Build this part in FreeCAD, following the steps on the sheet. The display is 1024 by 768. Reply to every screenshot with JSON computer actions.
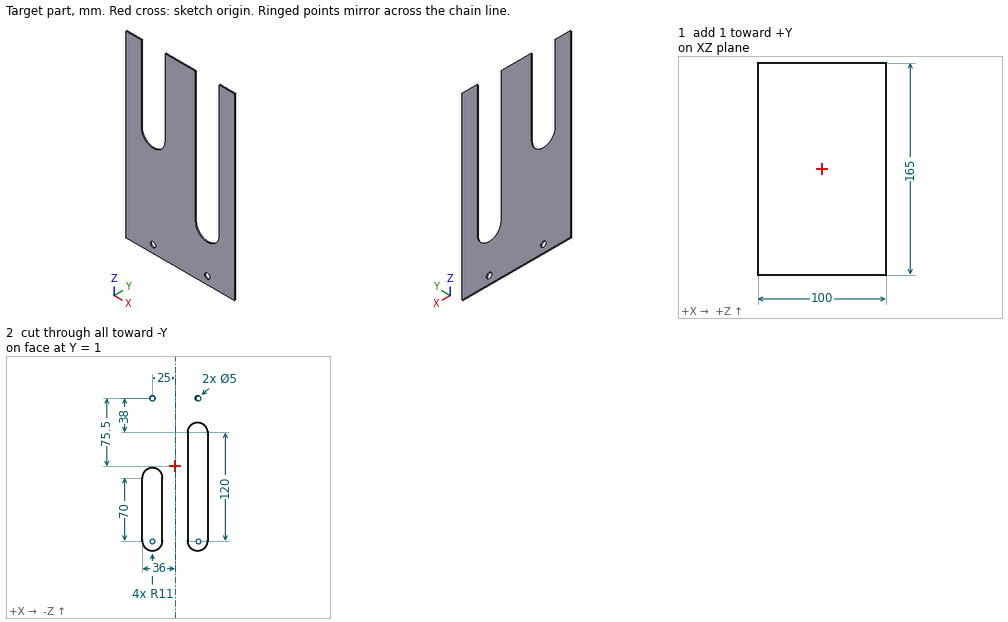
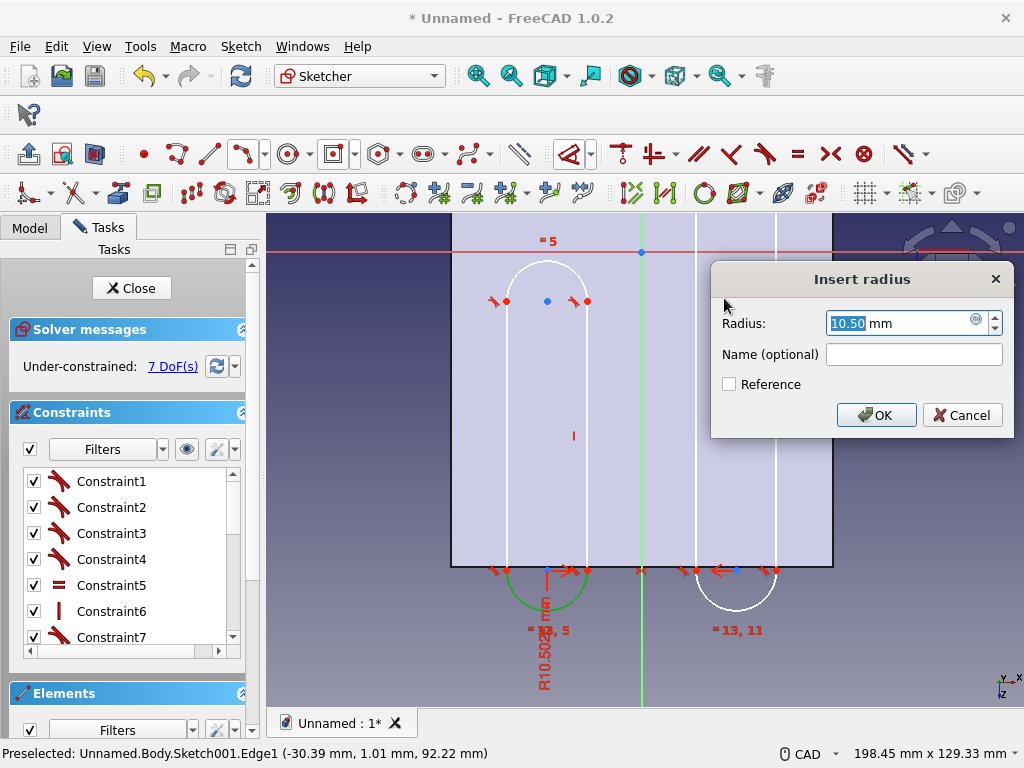
{"action": "type", "text": "11"}
{"action": "key", "text": "Return"}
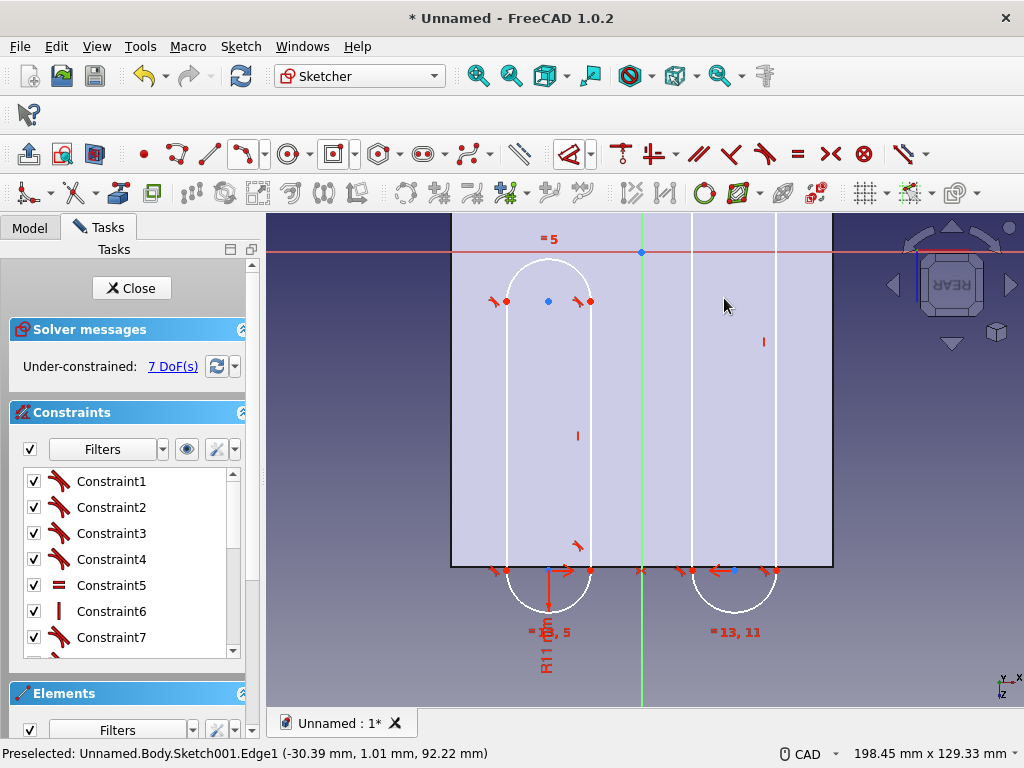
{"action": "scroll", "coordinate": [523, 605], "scroll_direction": "down", "scroll_amount": 4}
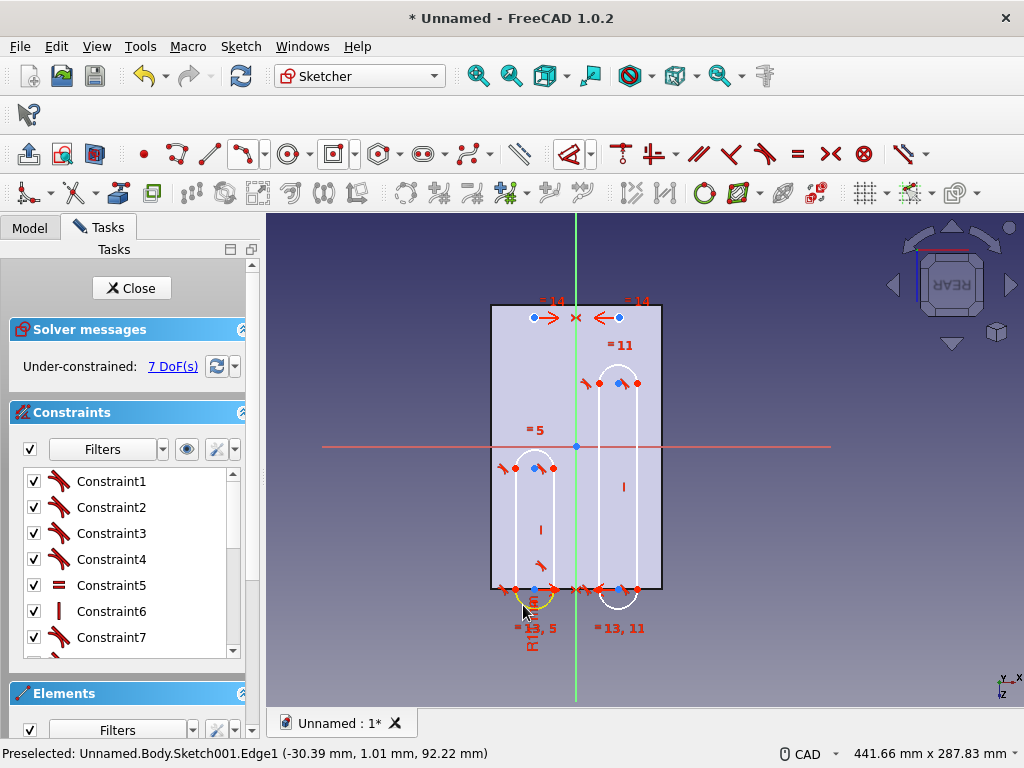
{"action": "scroll", "coordinate": [537, 315], "scroll_direction": "up", "scroll_amount": 8}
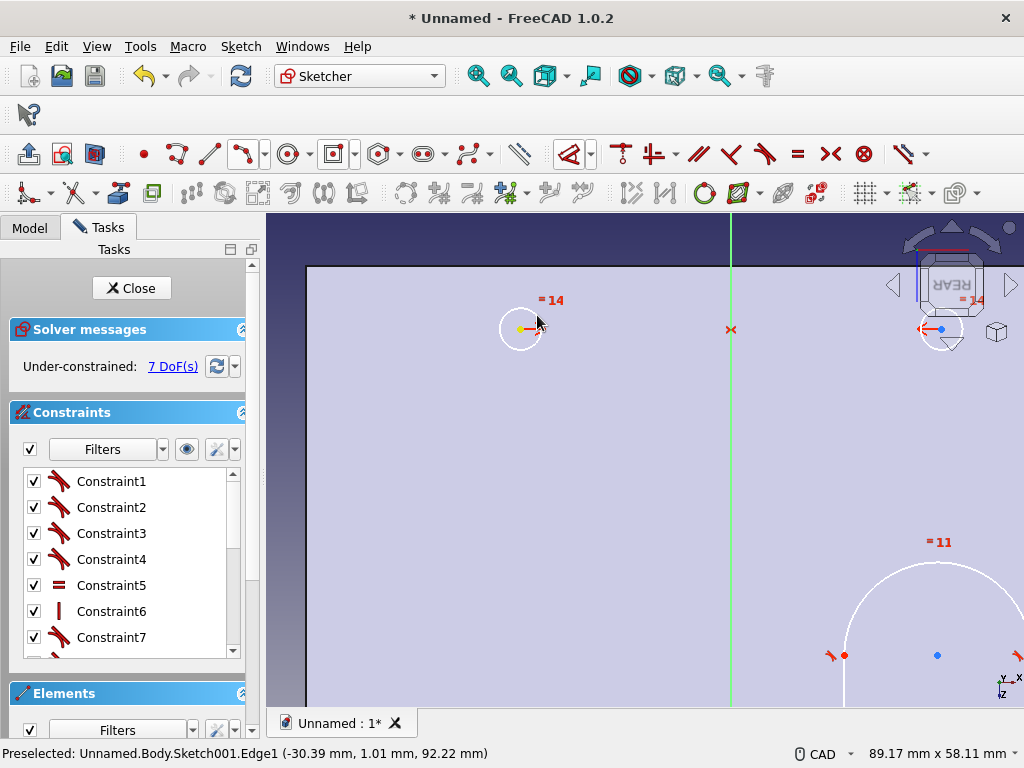
{"action": "left_click", "coordinate": [535, 314]}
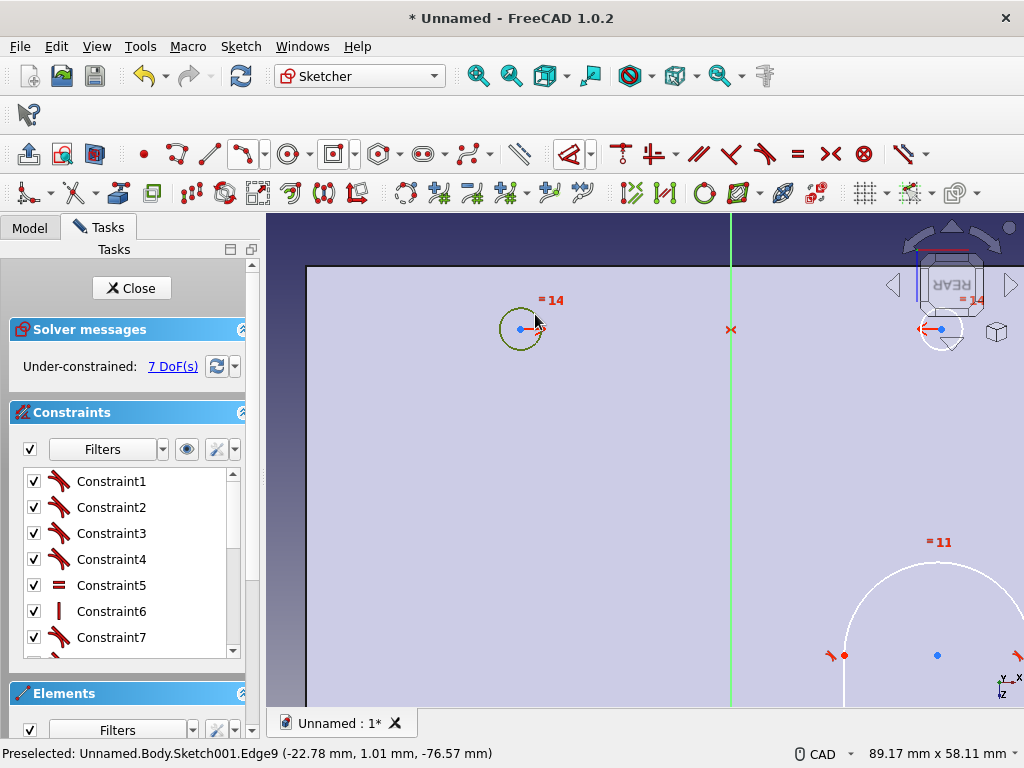
{"action": "key", "text": "k o"}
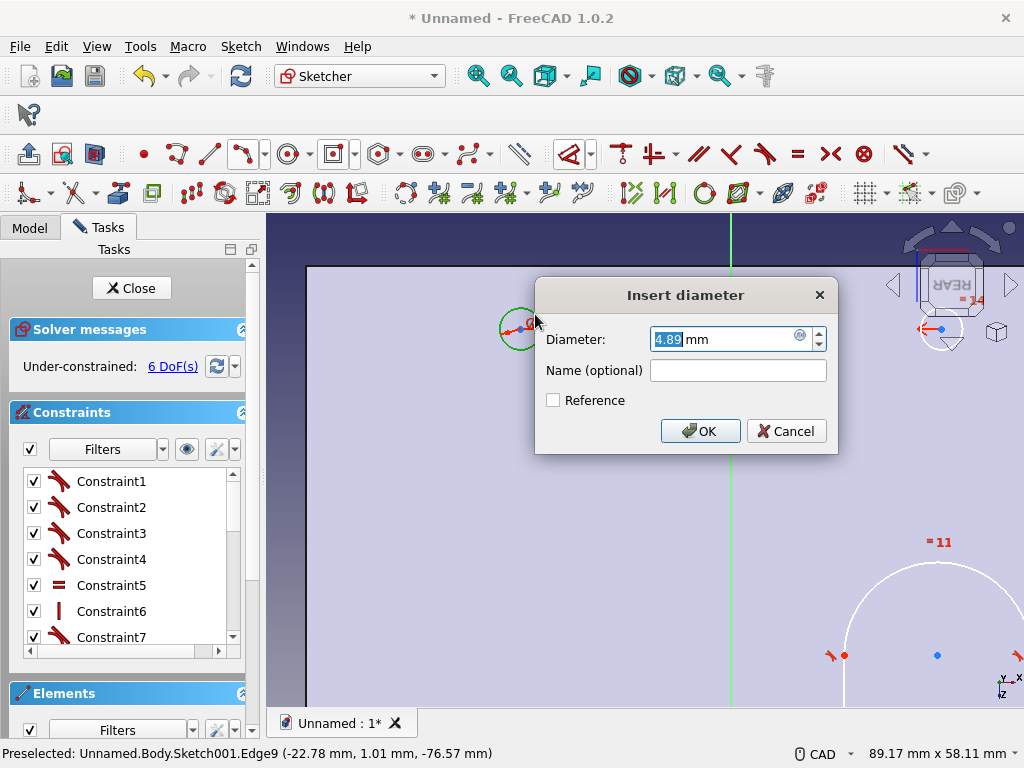
{"action": "type", "text": "5"}
{"action": "key", "text": "Return"}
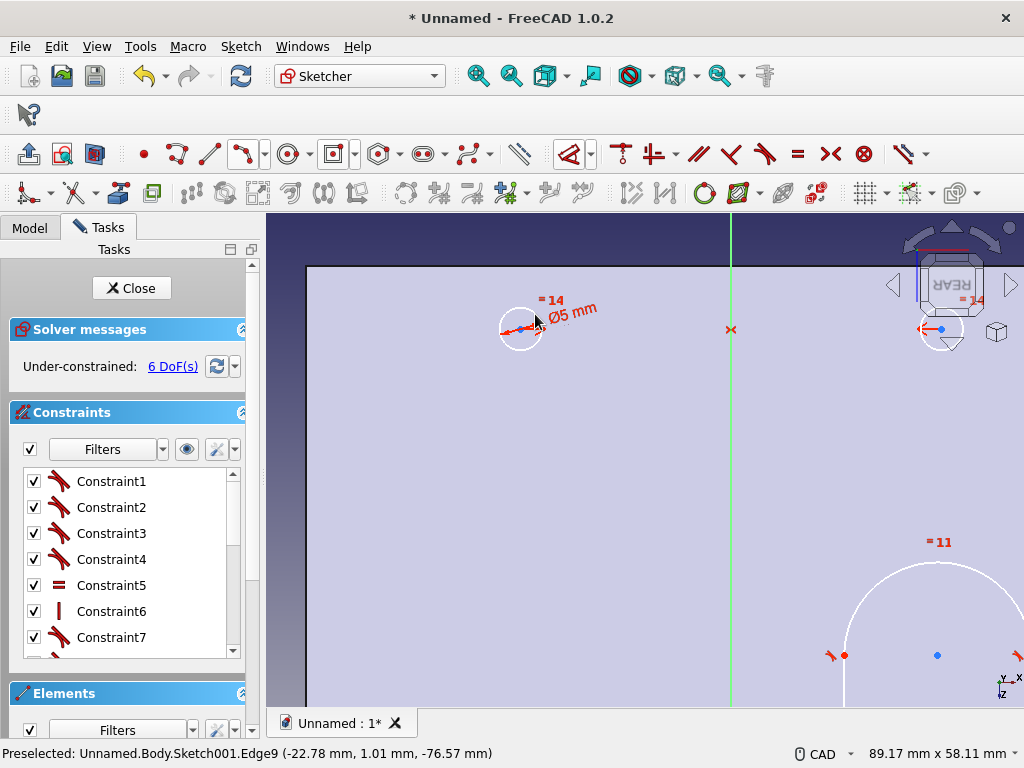
{"action": "scroll", "coordinate": [537, 315], "scroll_direction": "down", "scroll_amount": 8}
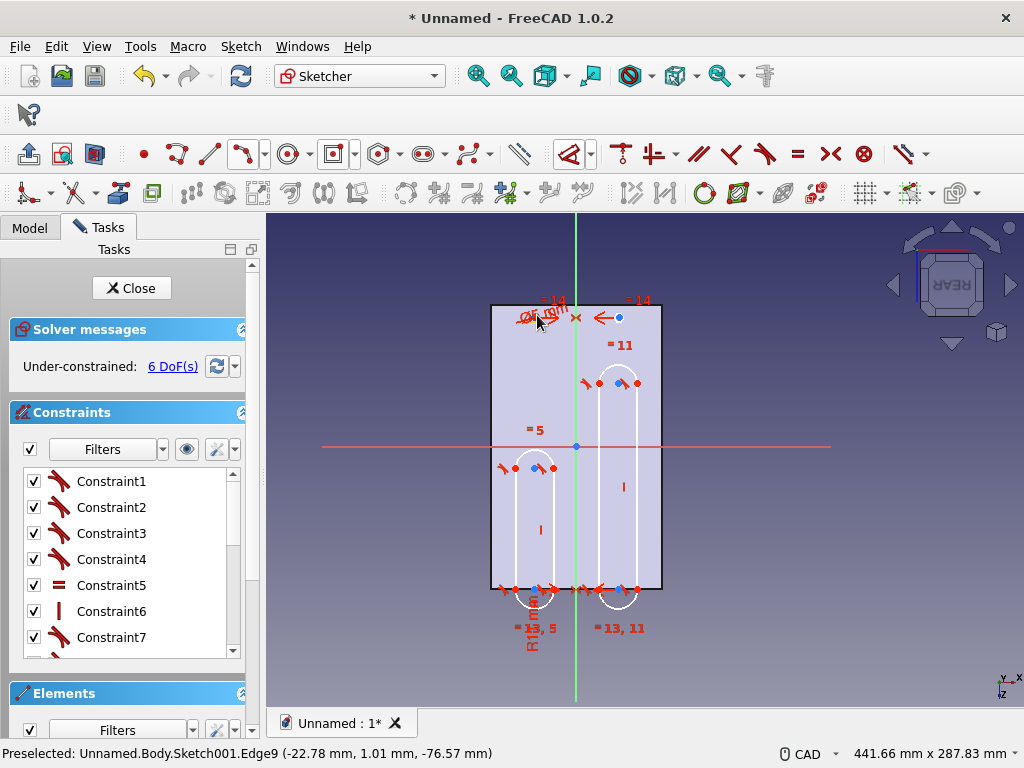
{"action": "left_click", "coordinate": [516, 554]}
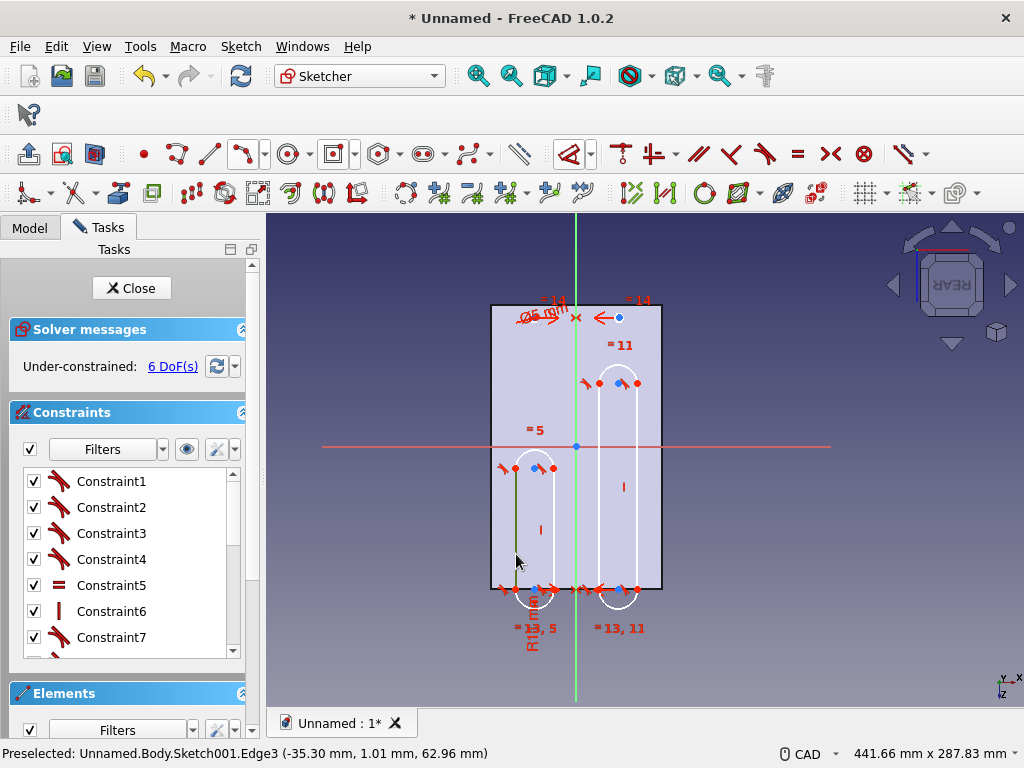
{"action": "key", "text": "i"}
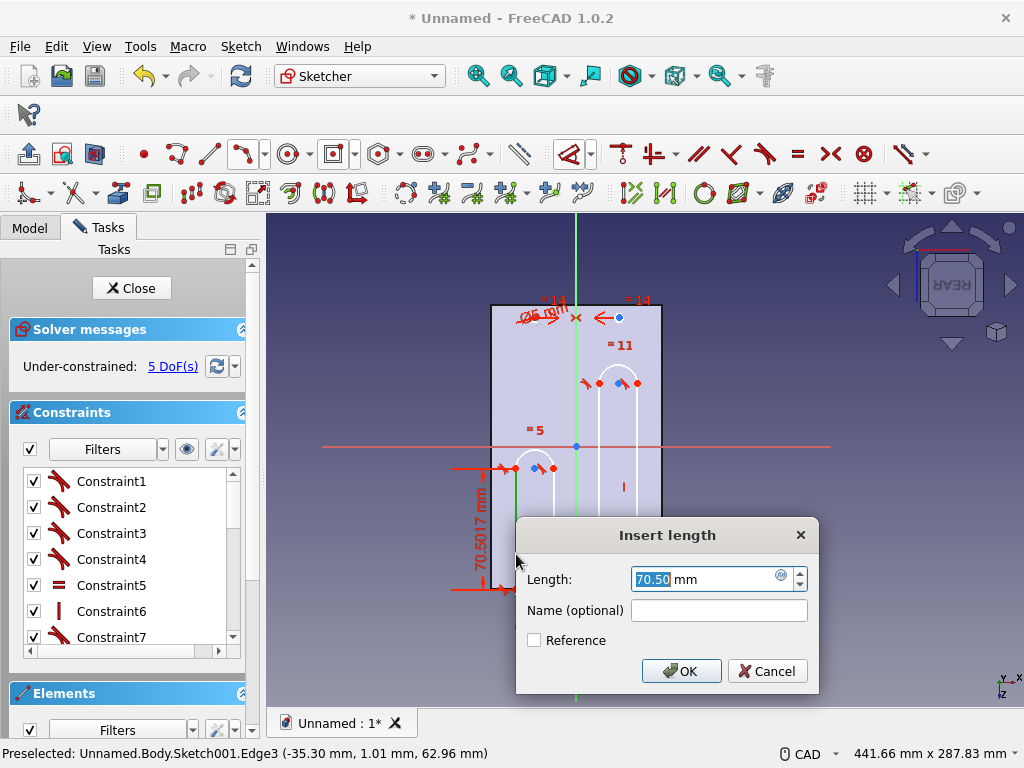
{"action": "type", "text": "70"}
{"action": "key", "text": "Return"}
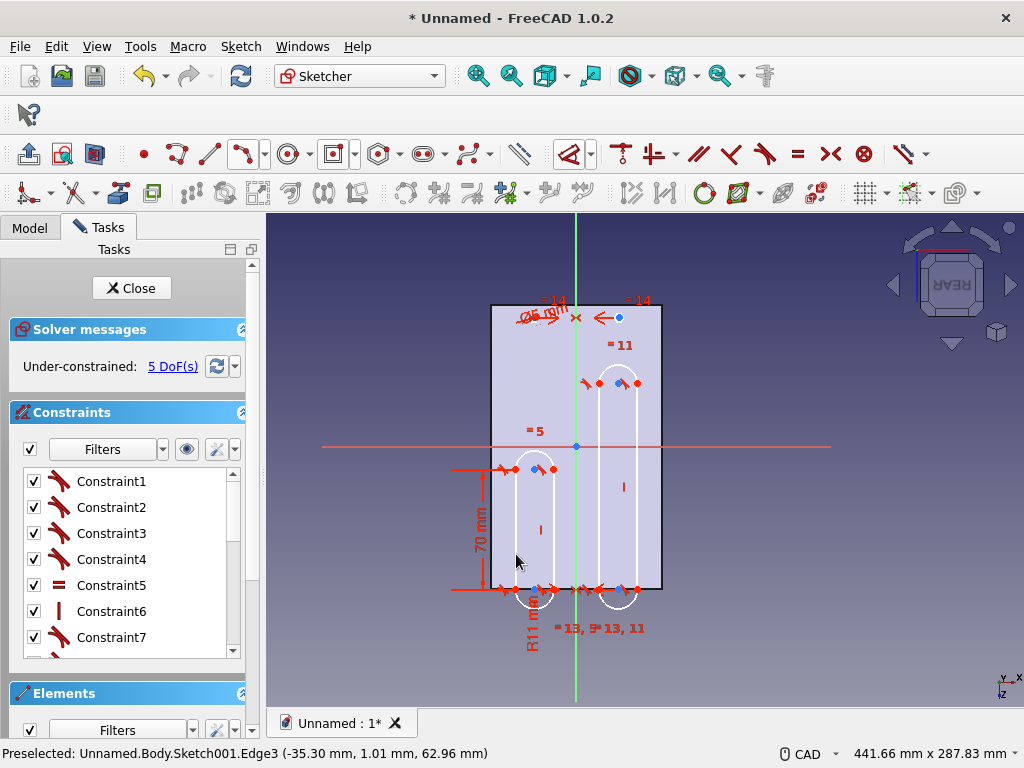
{"action": "left_click", "coordinate": [534, 318]}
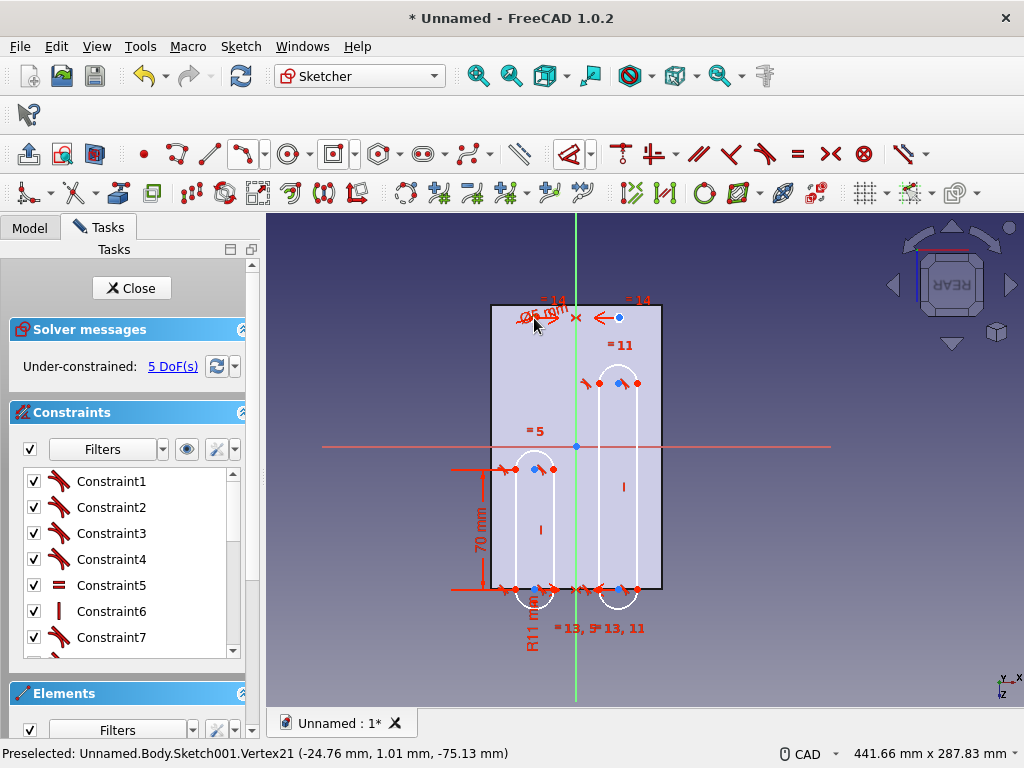
{"action": "left_click", "coordinate": [590, 154]}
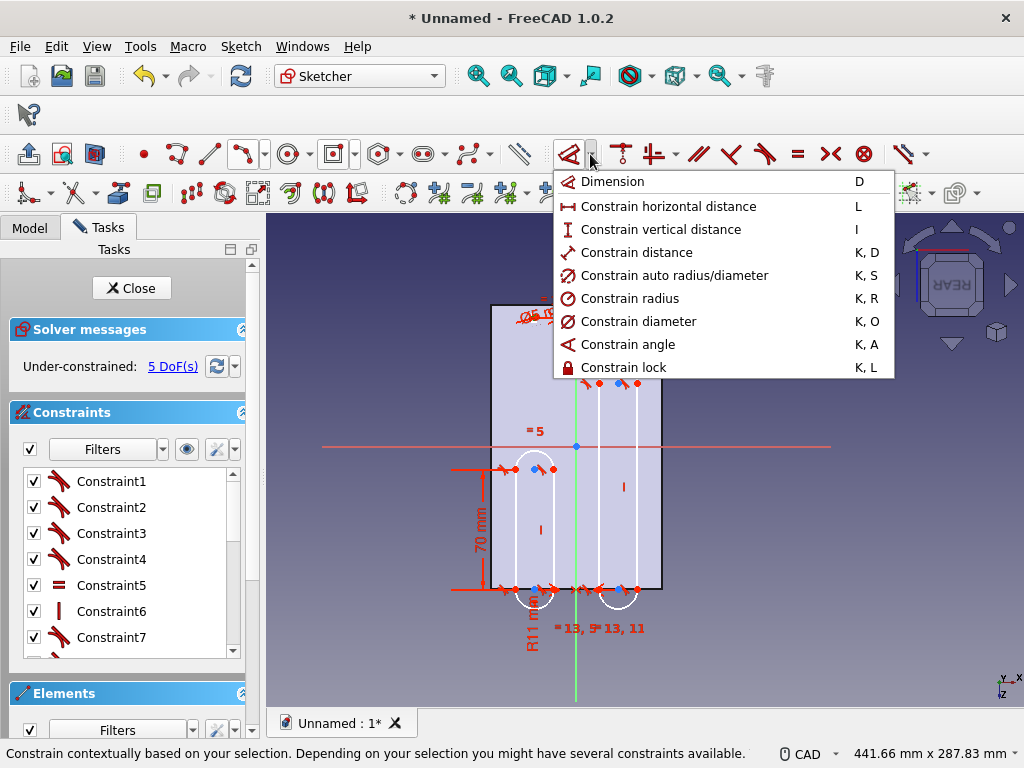
{"action": "left_click", "coordinate": [724, 206]}